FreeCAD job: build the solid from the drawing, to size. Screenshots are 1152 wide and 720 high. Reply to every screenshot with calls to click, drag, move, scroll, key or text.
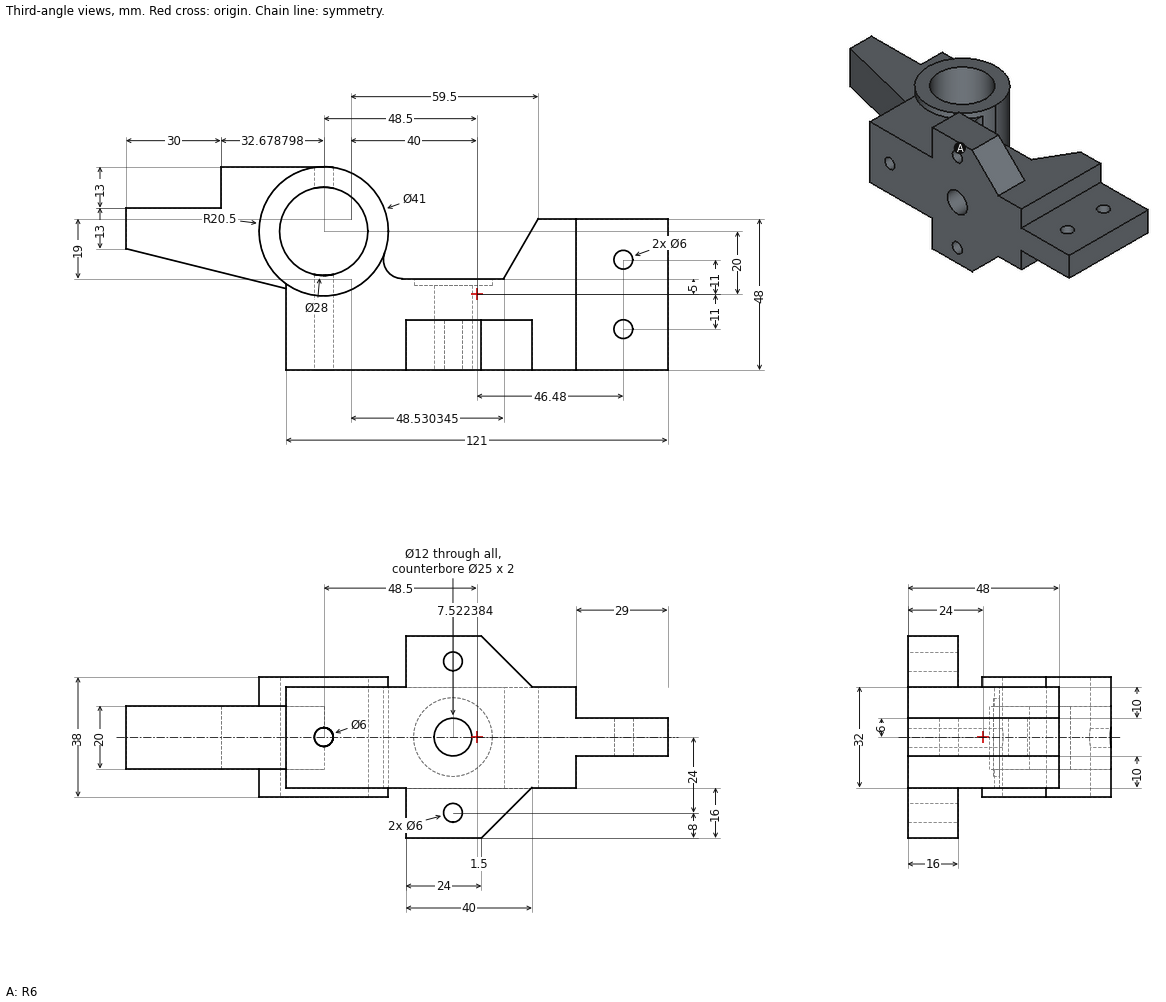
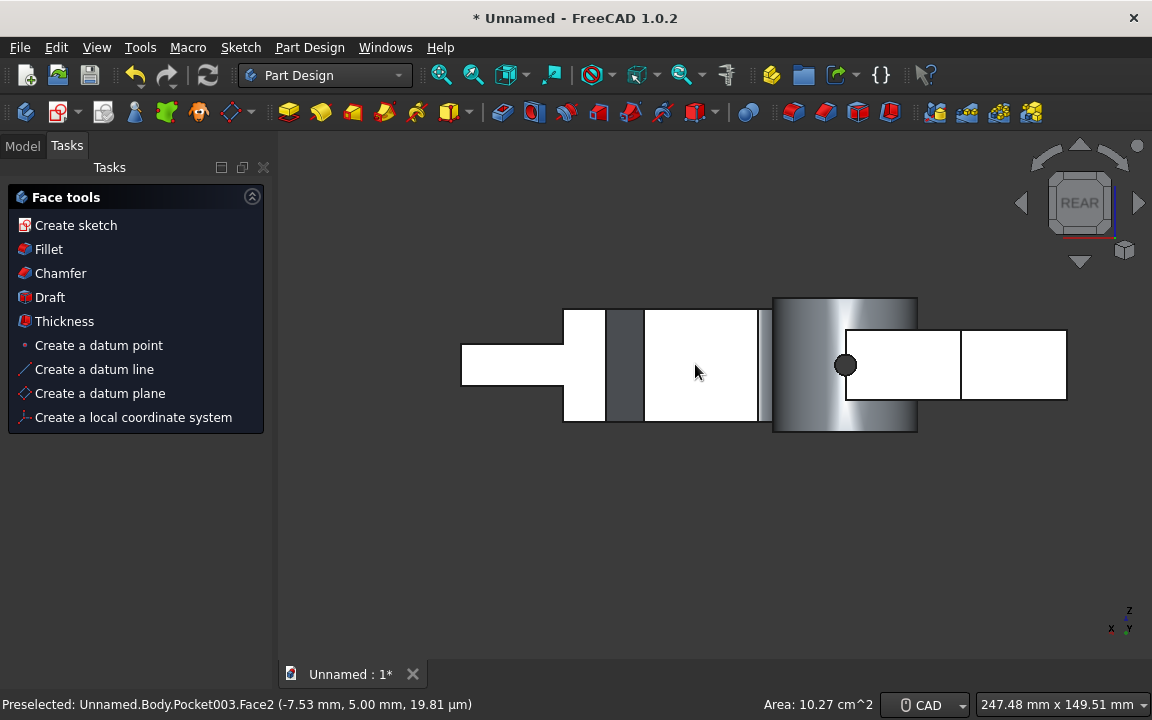
click(58, 112)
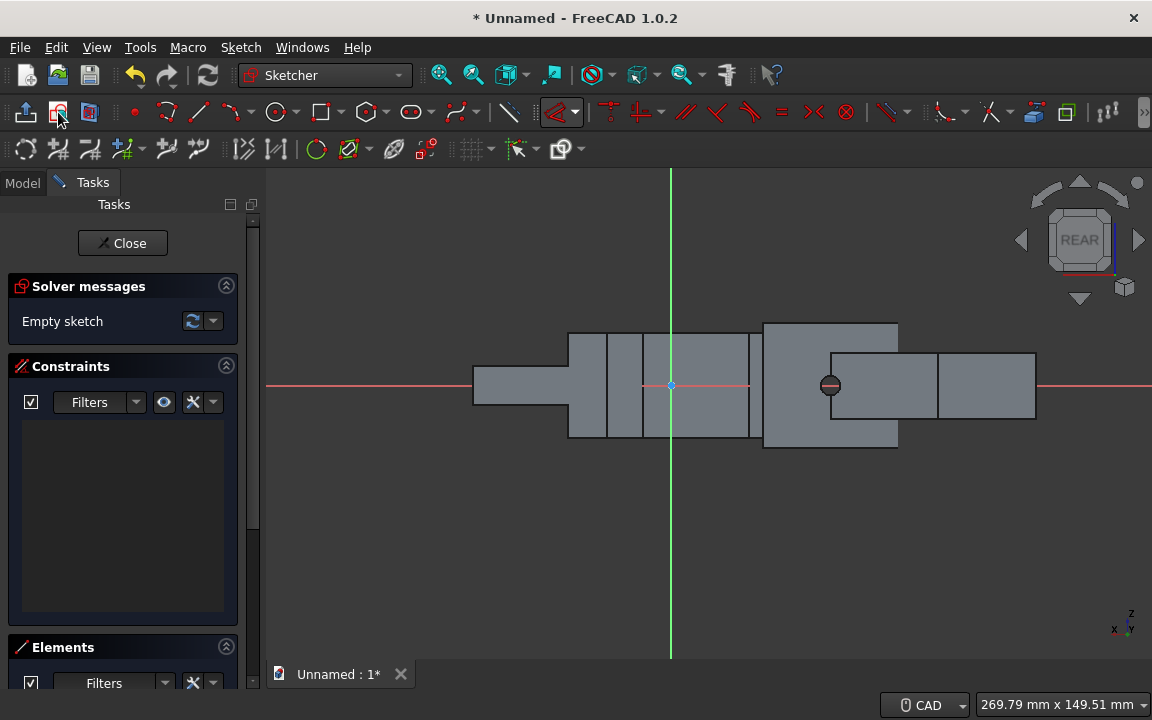
scroll(702, 381, up, 10)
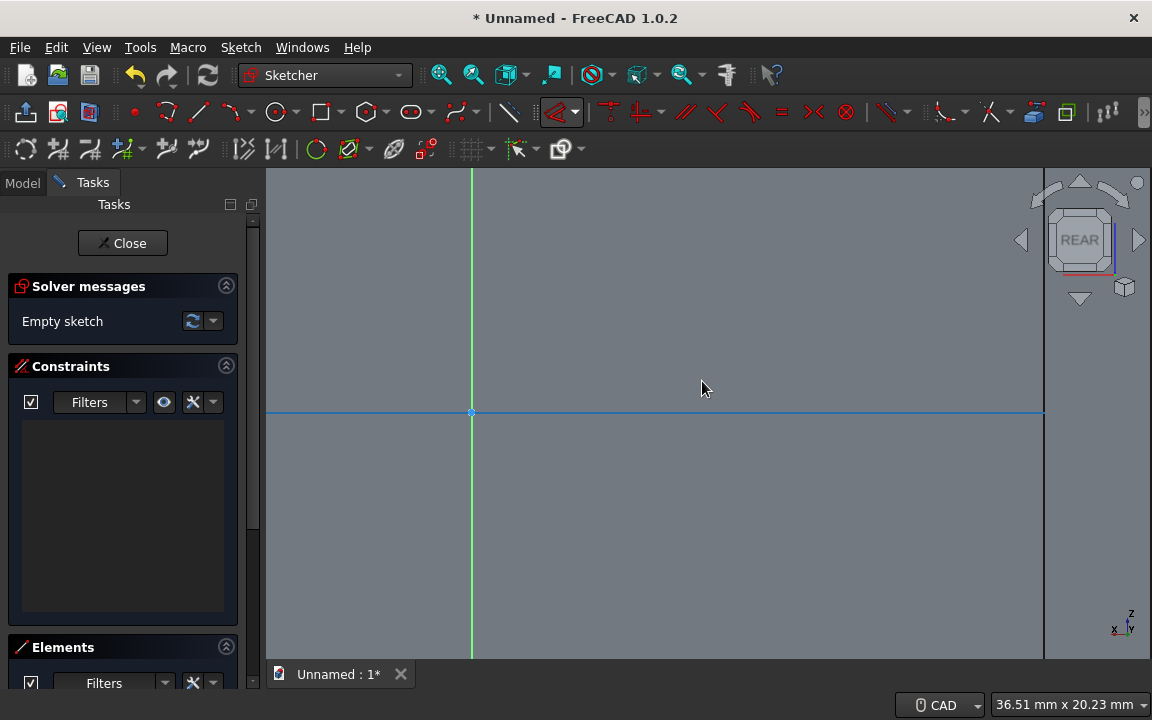
key(g)
key(c)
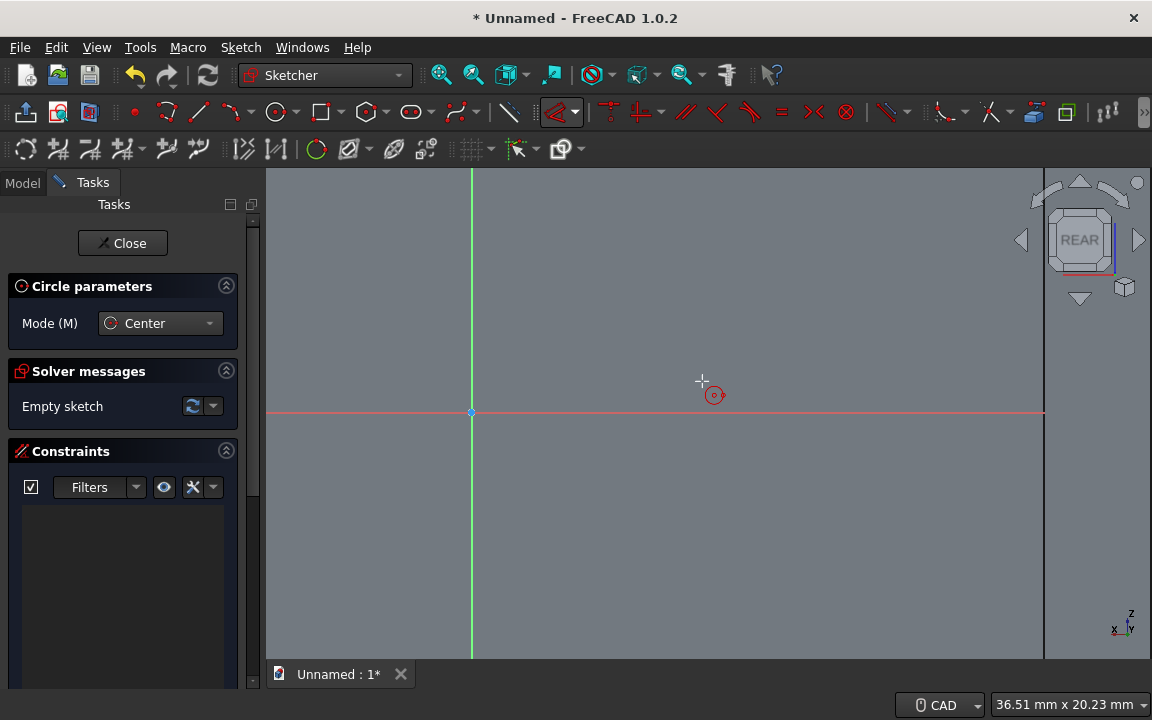
click(654, 413)
move(757, 310)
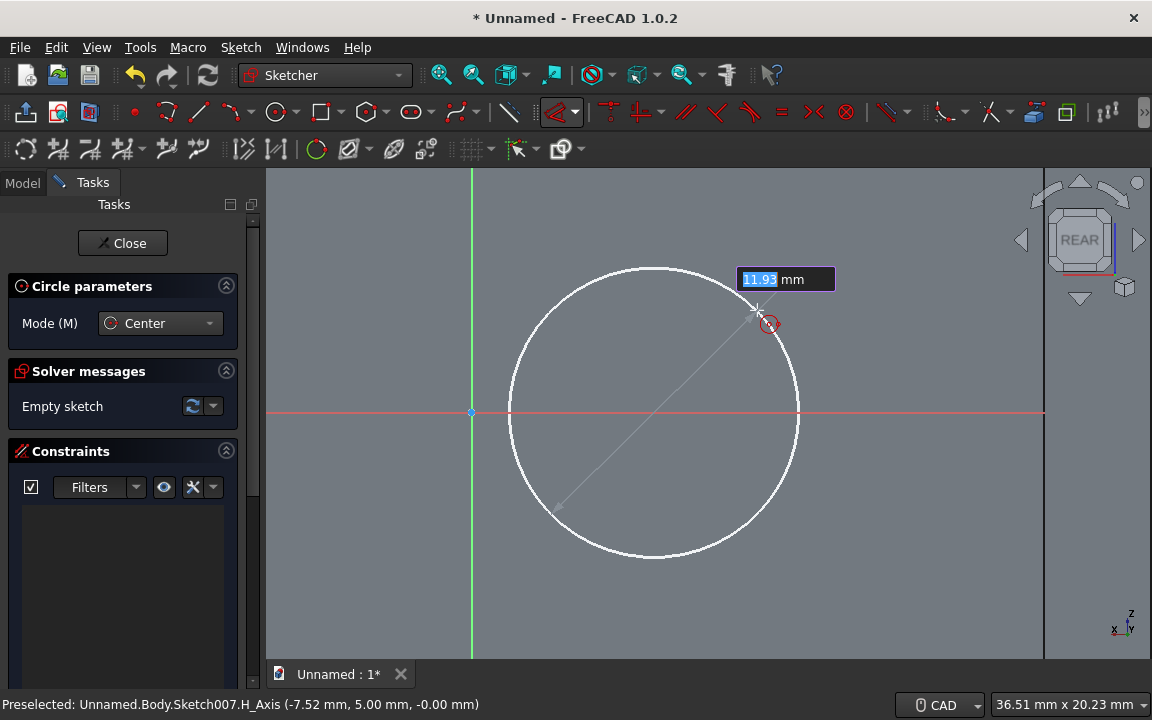
text(12)
key(Return)
key(Escape)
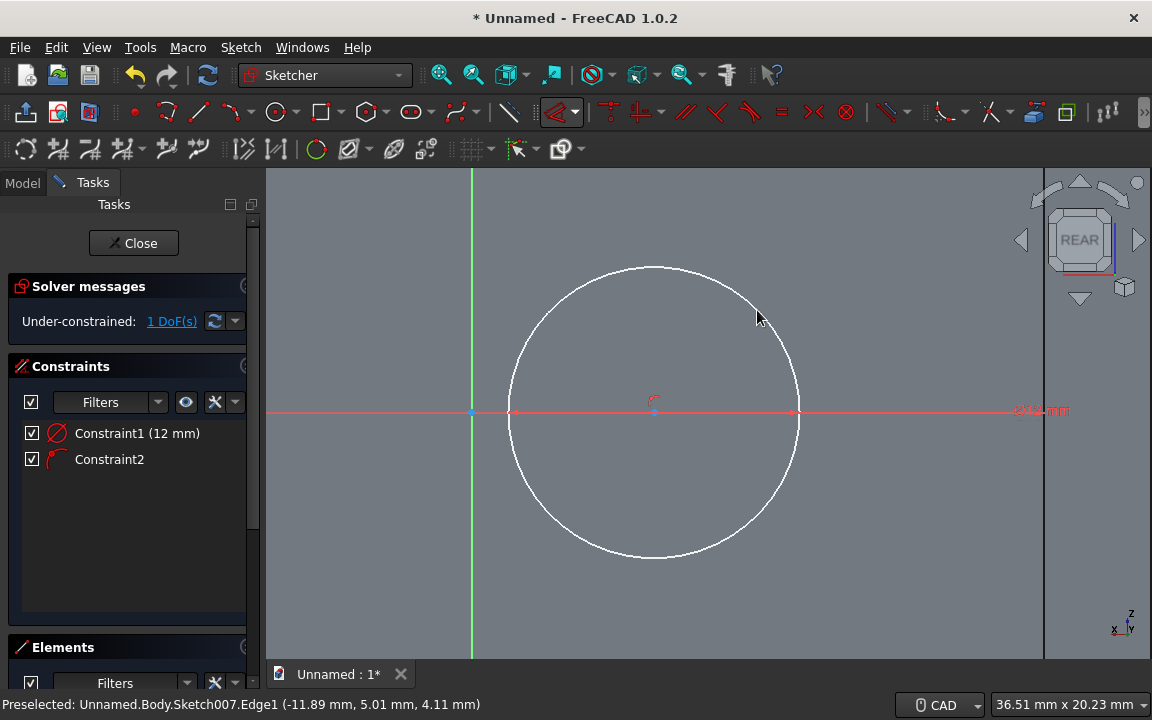
click(654, 413)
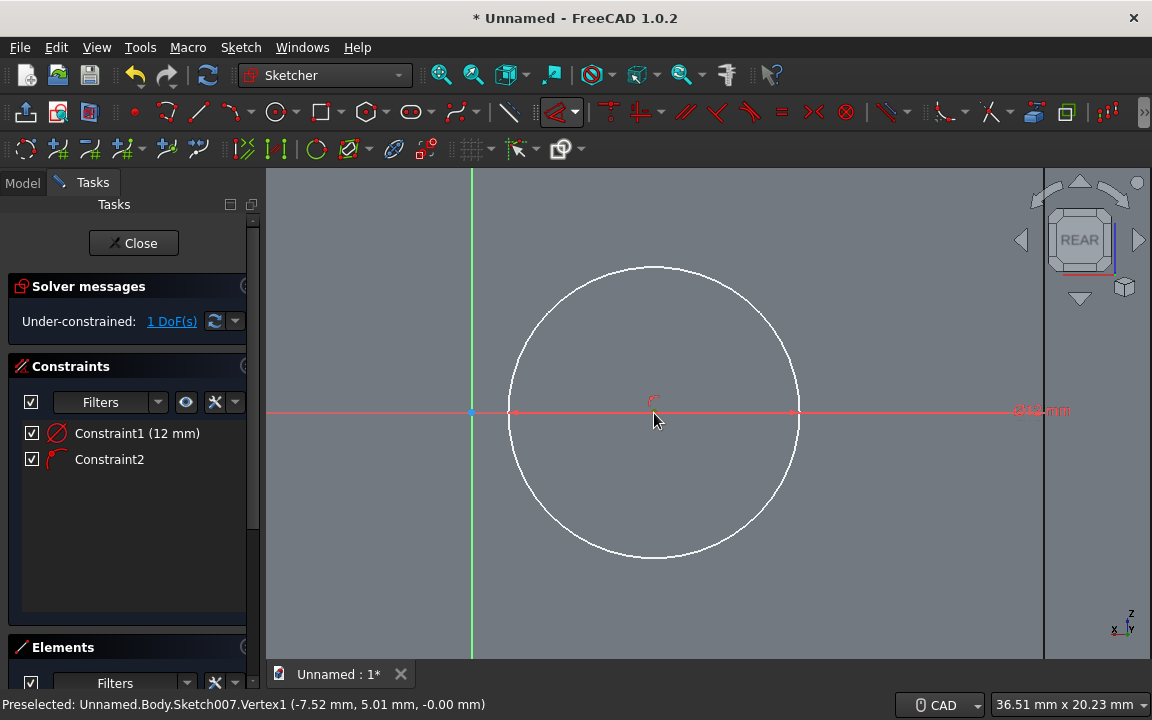
key(l)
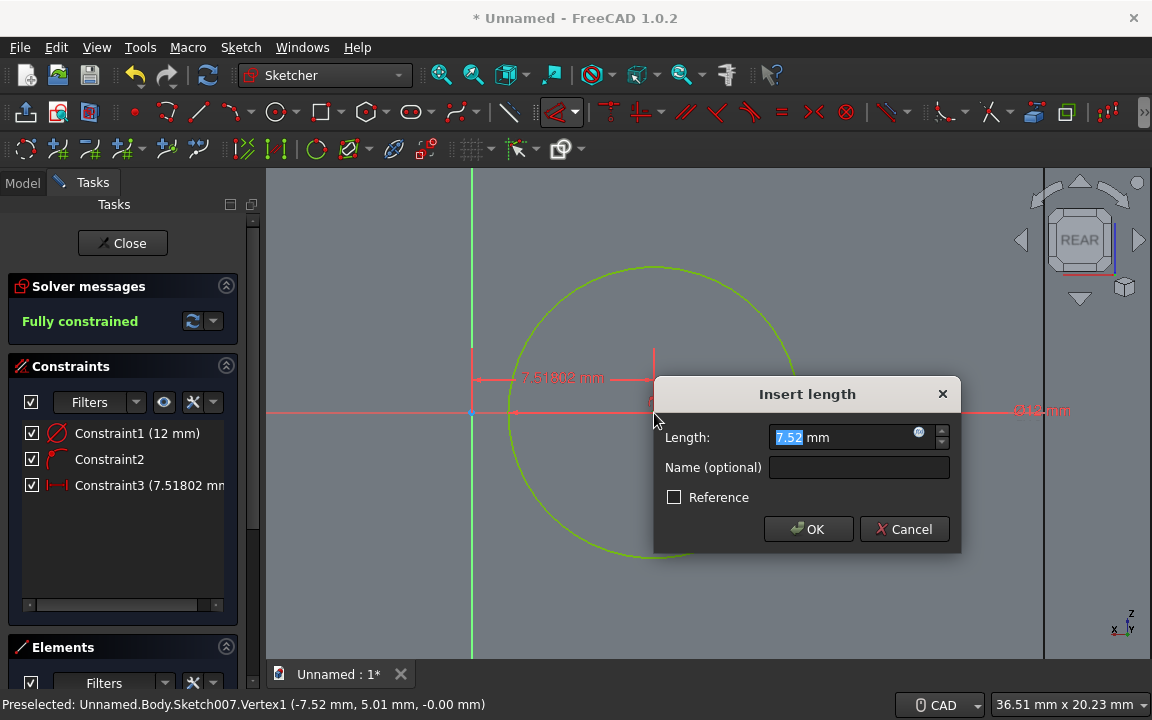
text(7.522384)
key(Return)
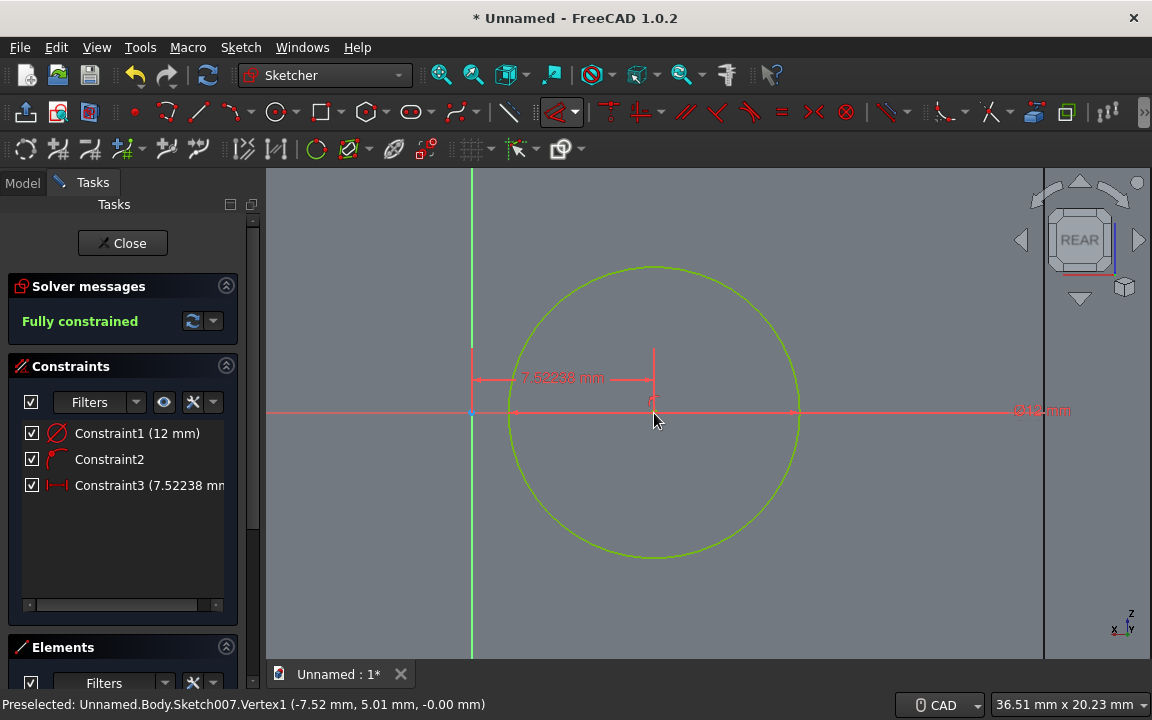
click(123, 243)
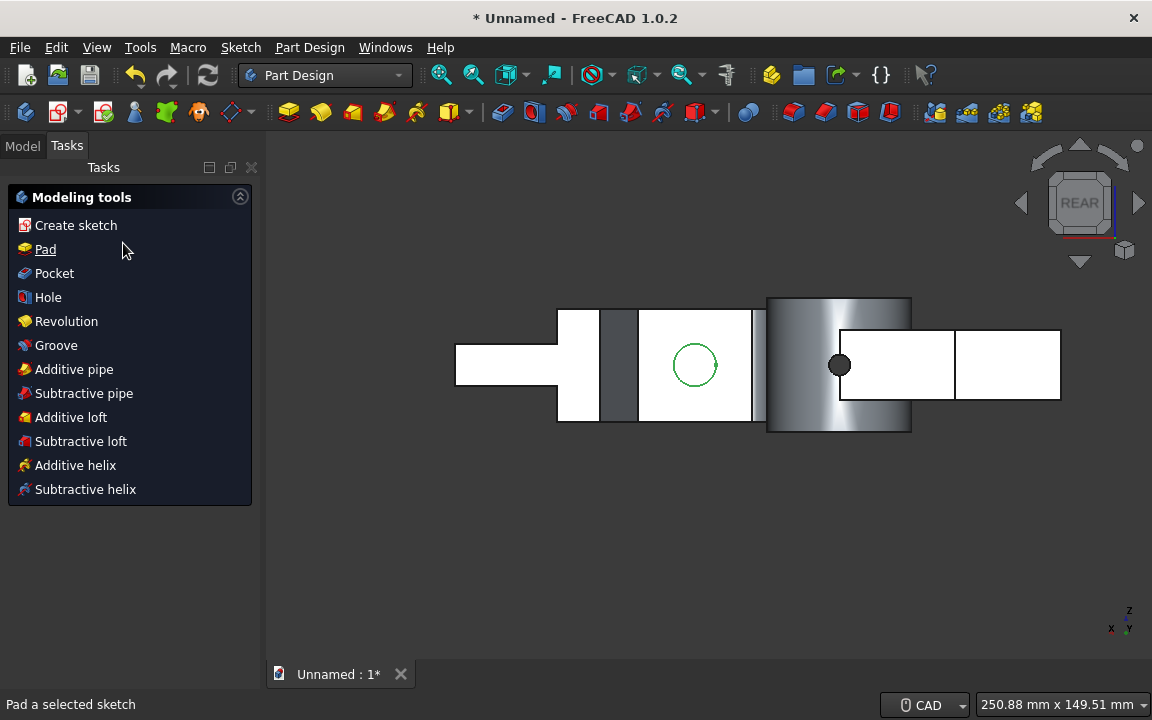
click(536, 112)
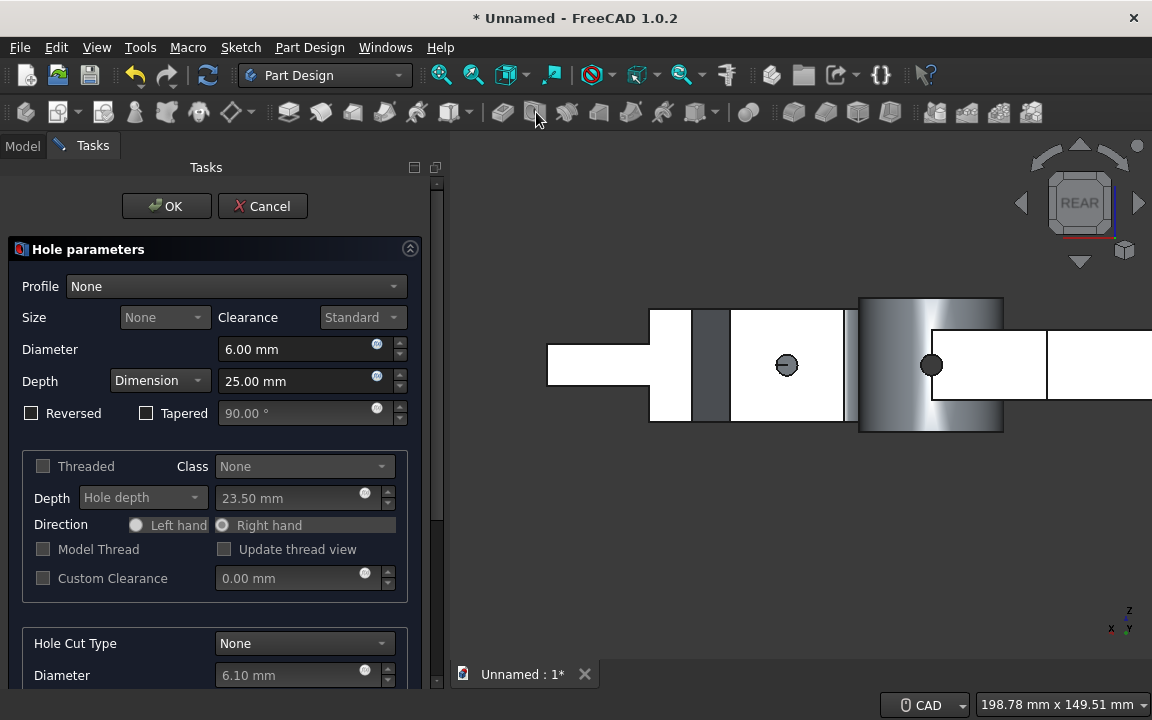
triple_click(305, 349)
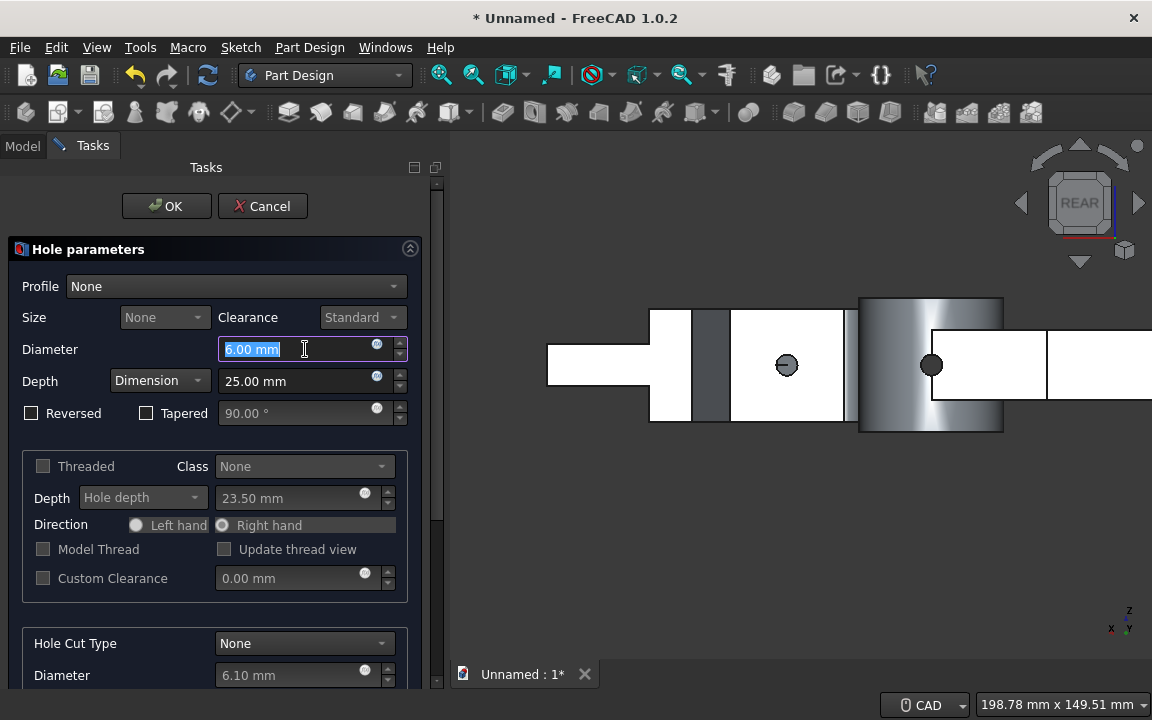
text(12)
key(Tab)